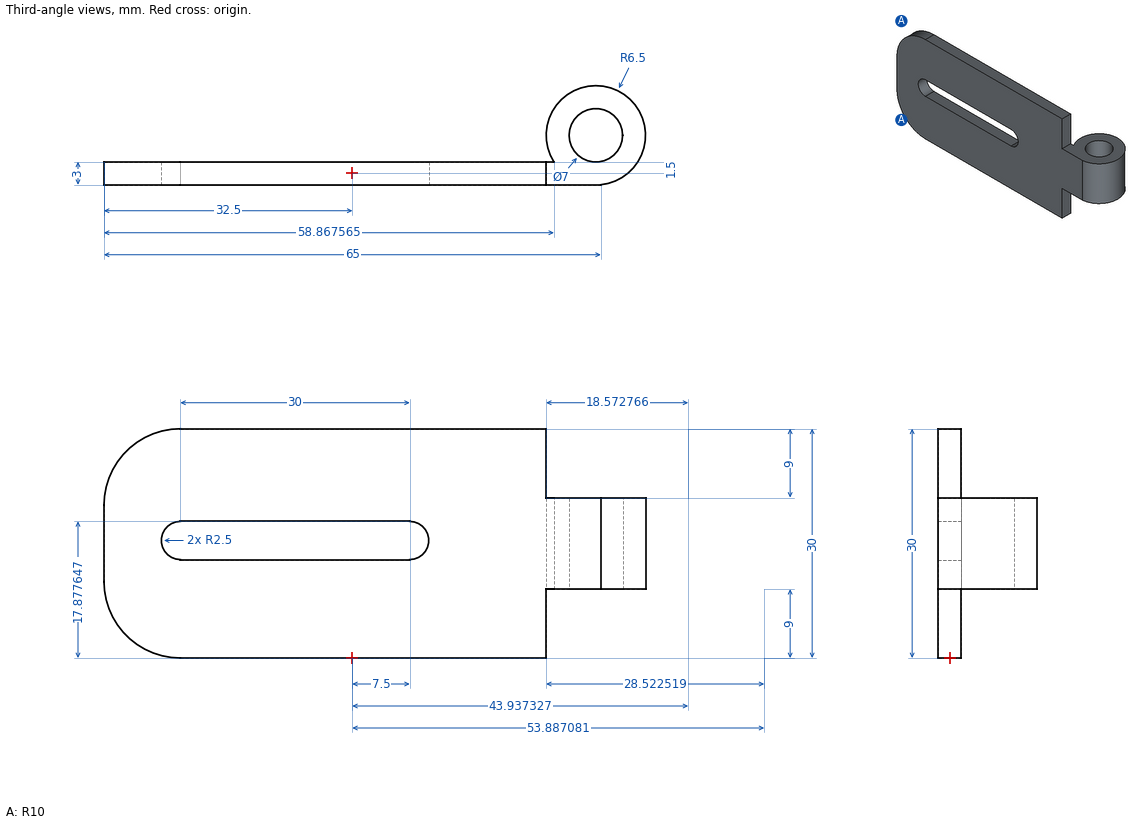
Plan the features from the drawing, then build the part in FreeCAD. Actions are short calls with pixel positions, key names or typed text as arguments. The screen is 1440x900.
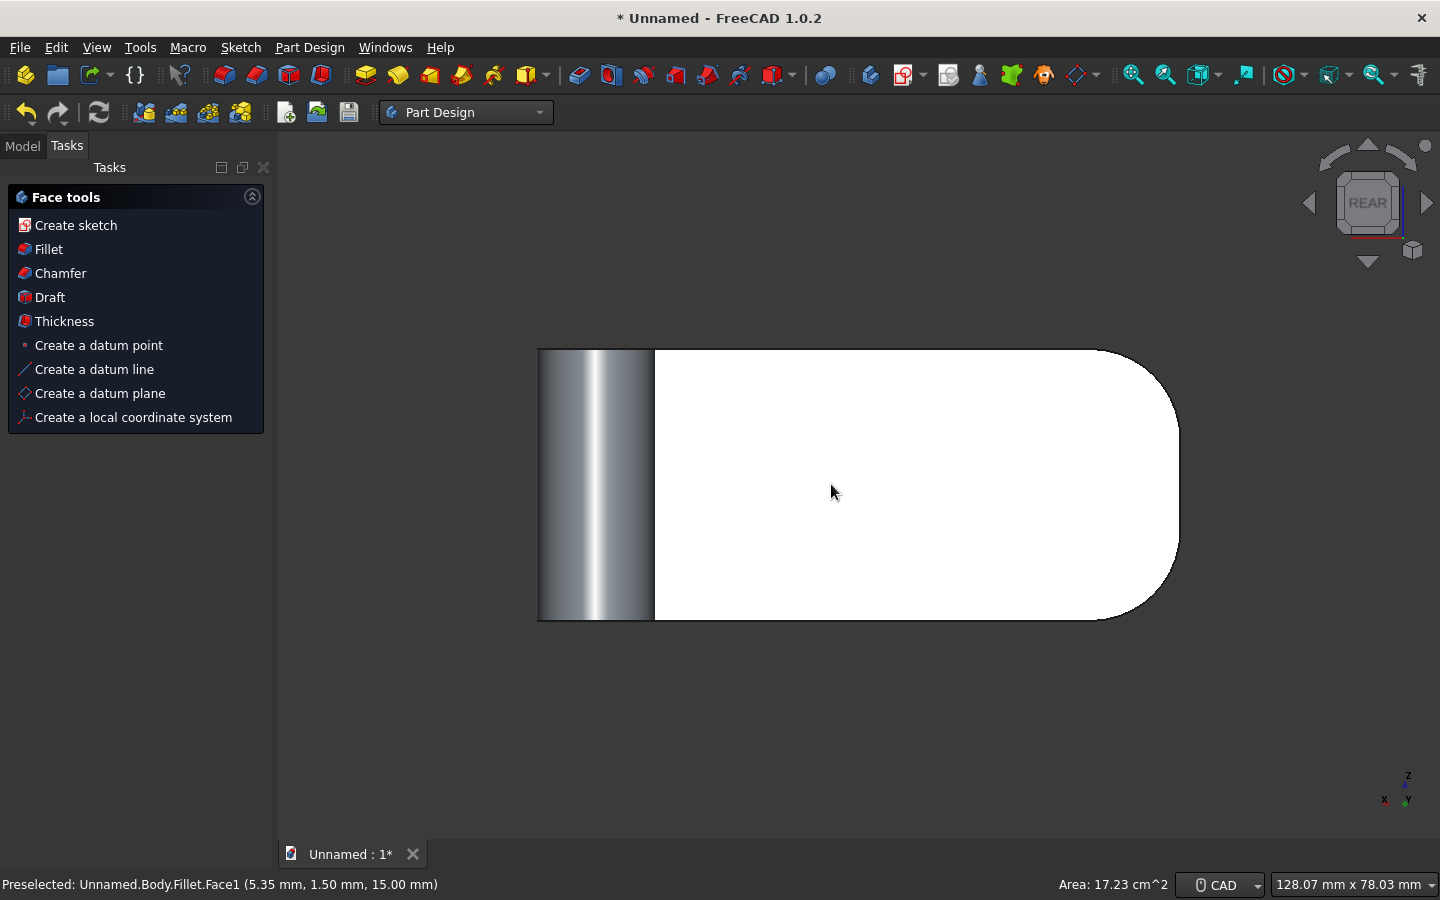
click(904, 76)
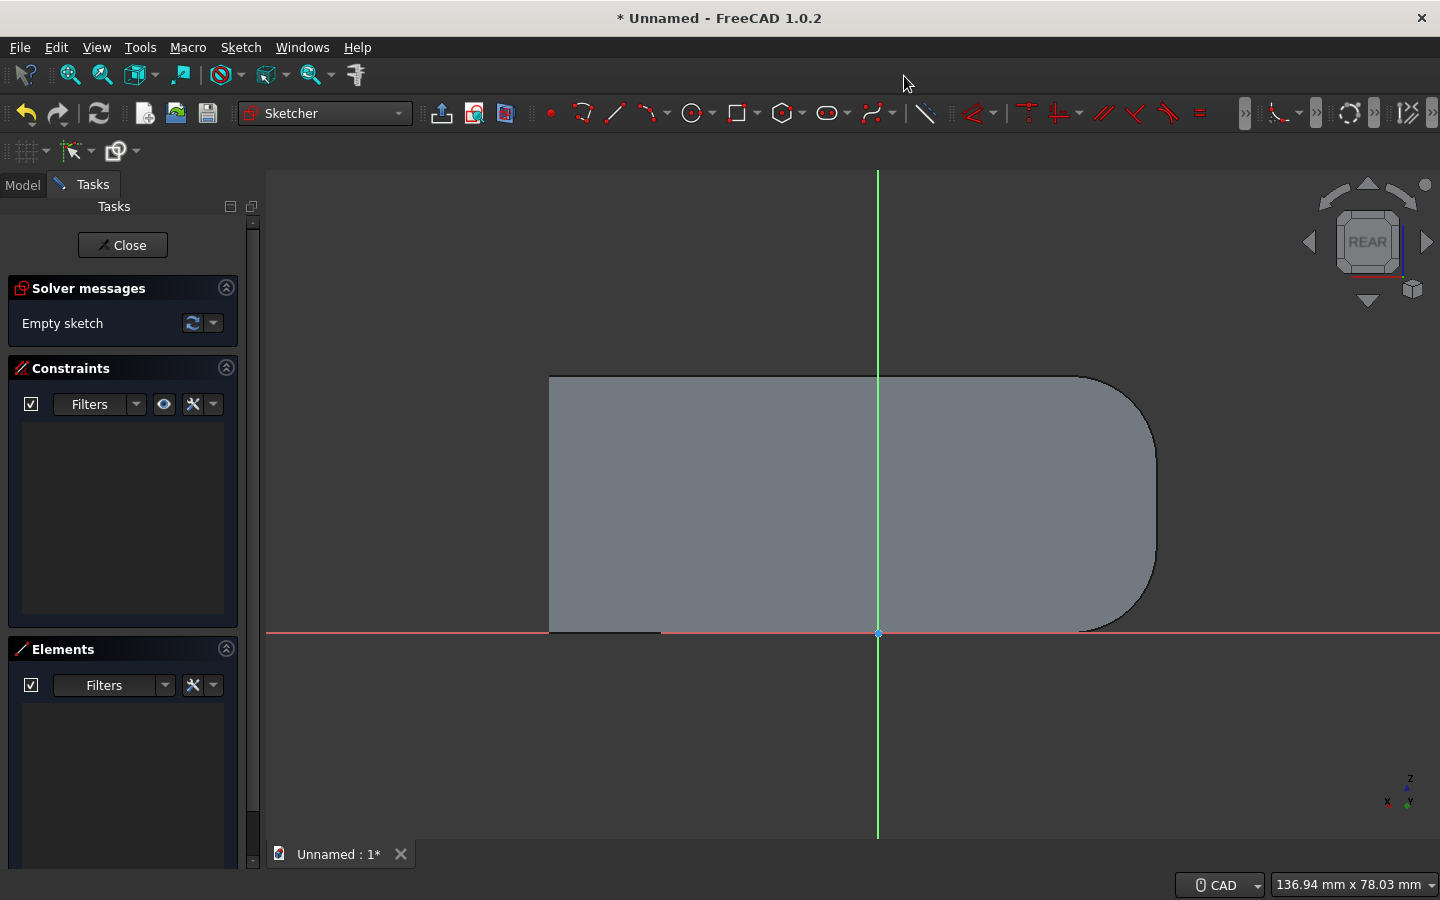
click(506, 114)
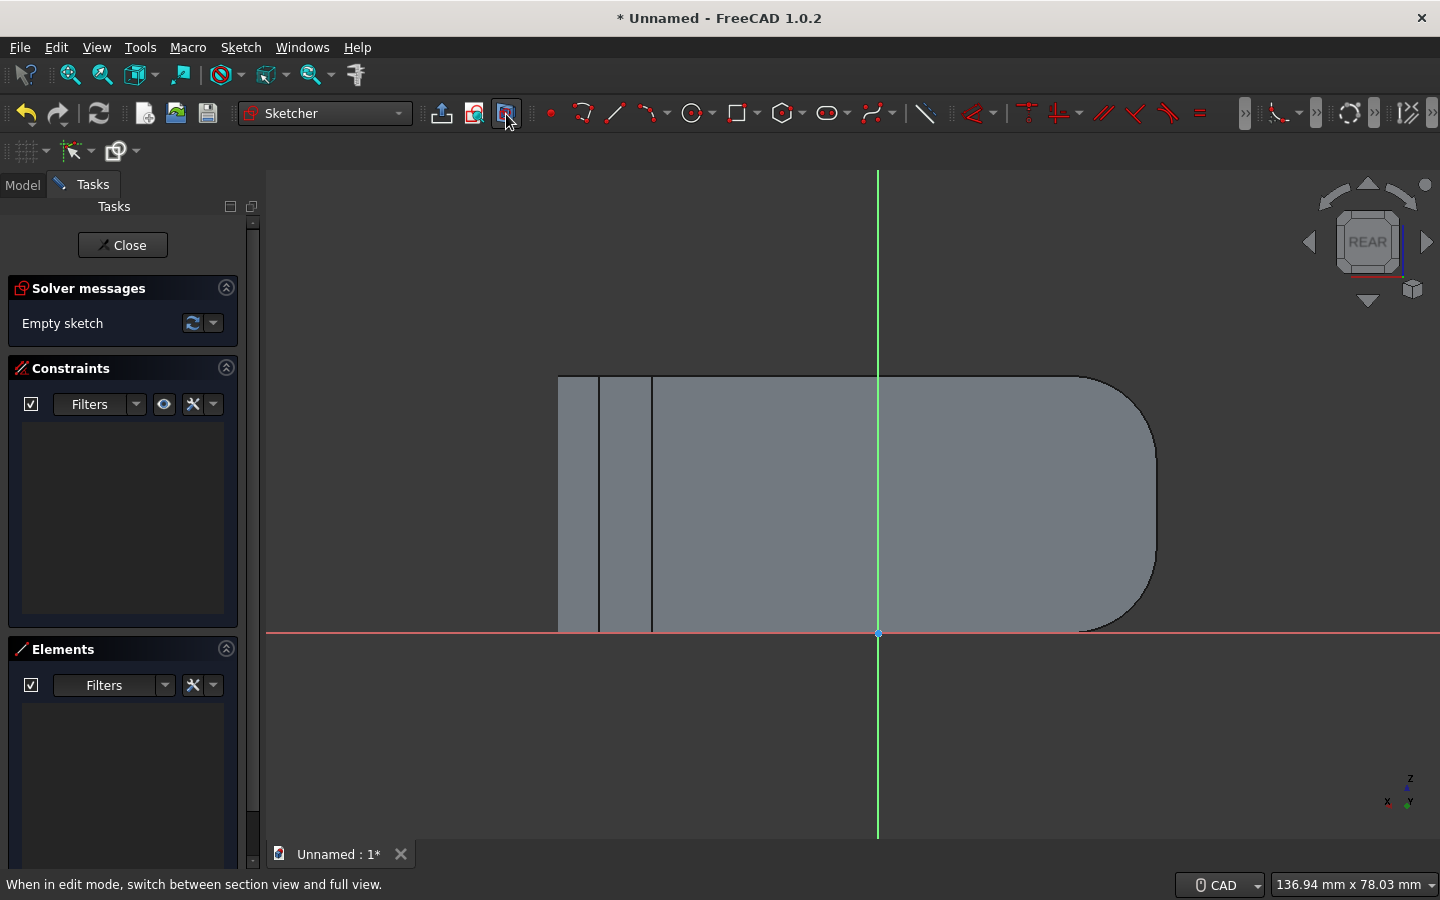
scroll(1071, 599, up, 4)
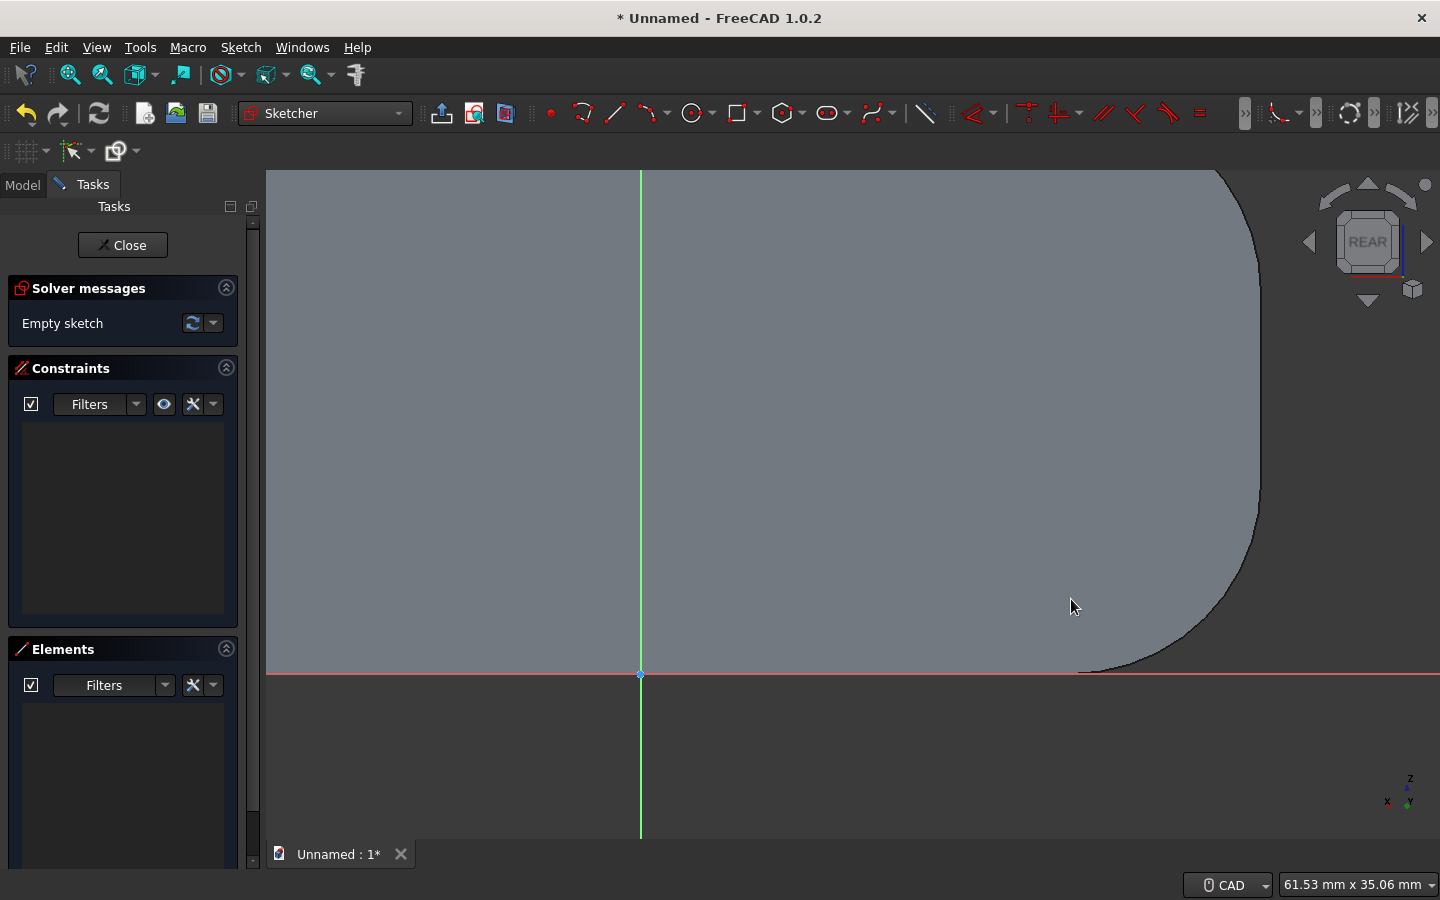
click(828, 114)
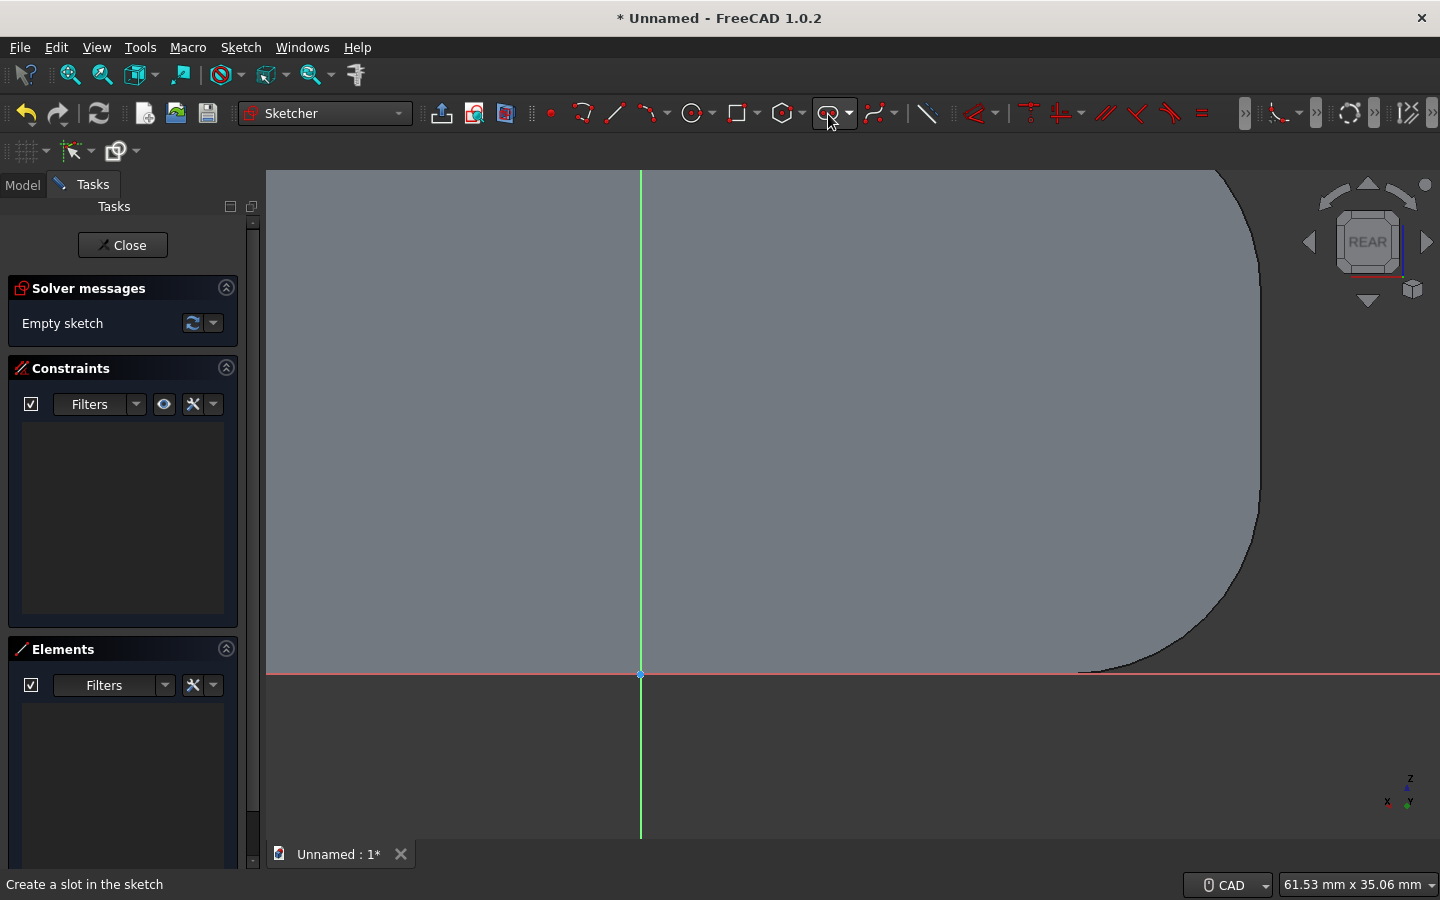
click(498, 381)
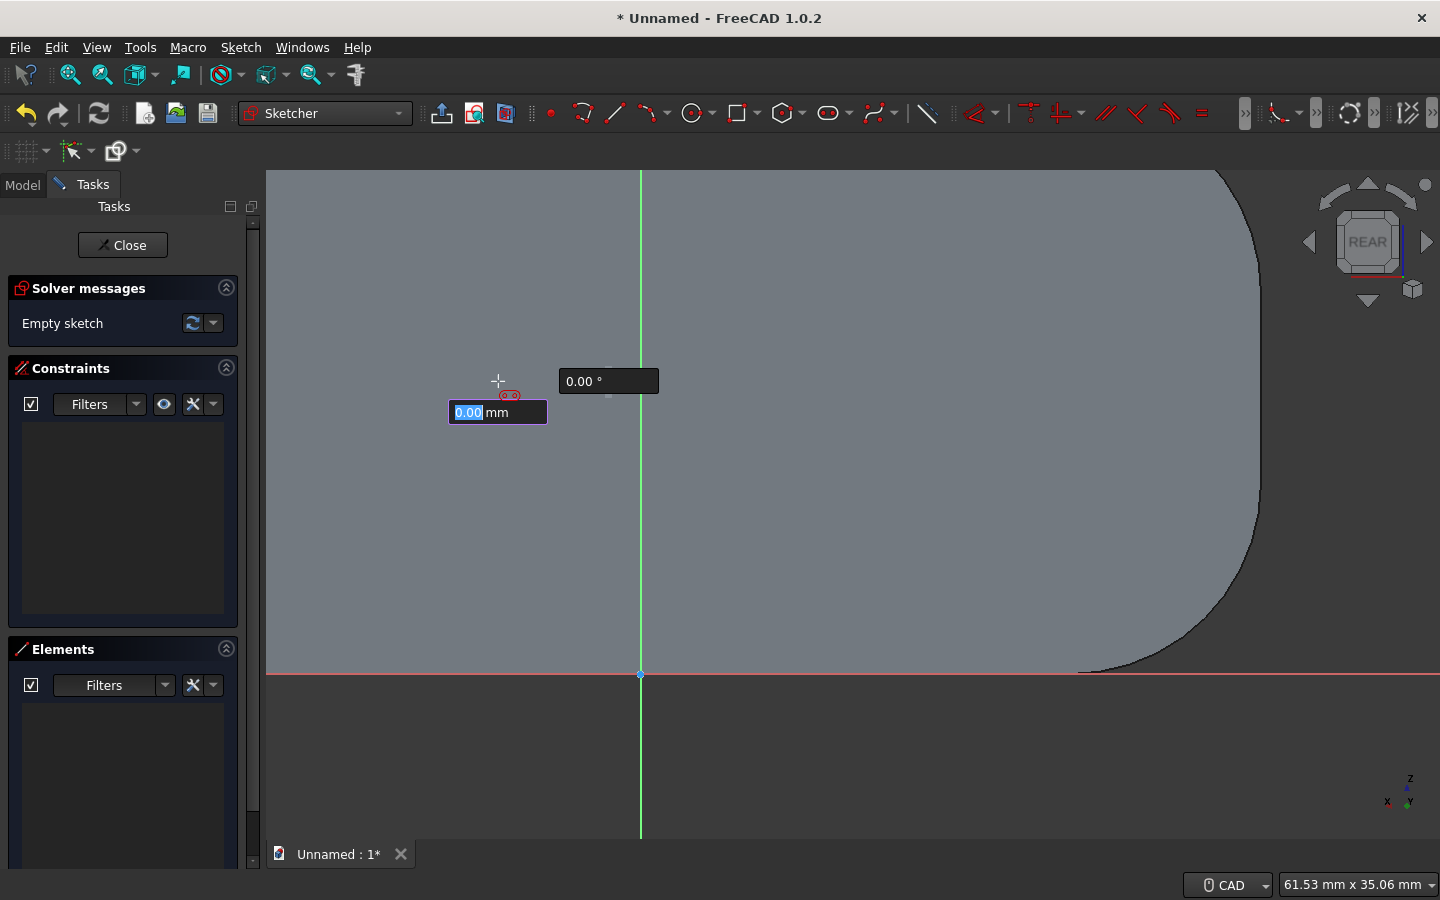
click(1070, 381)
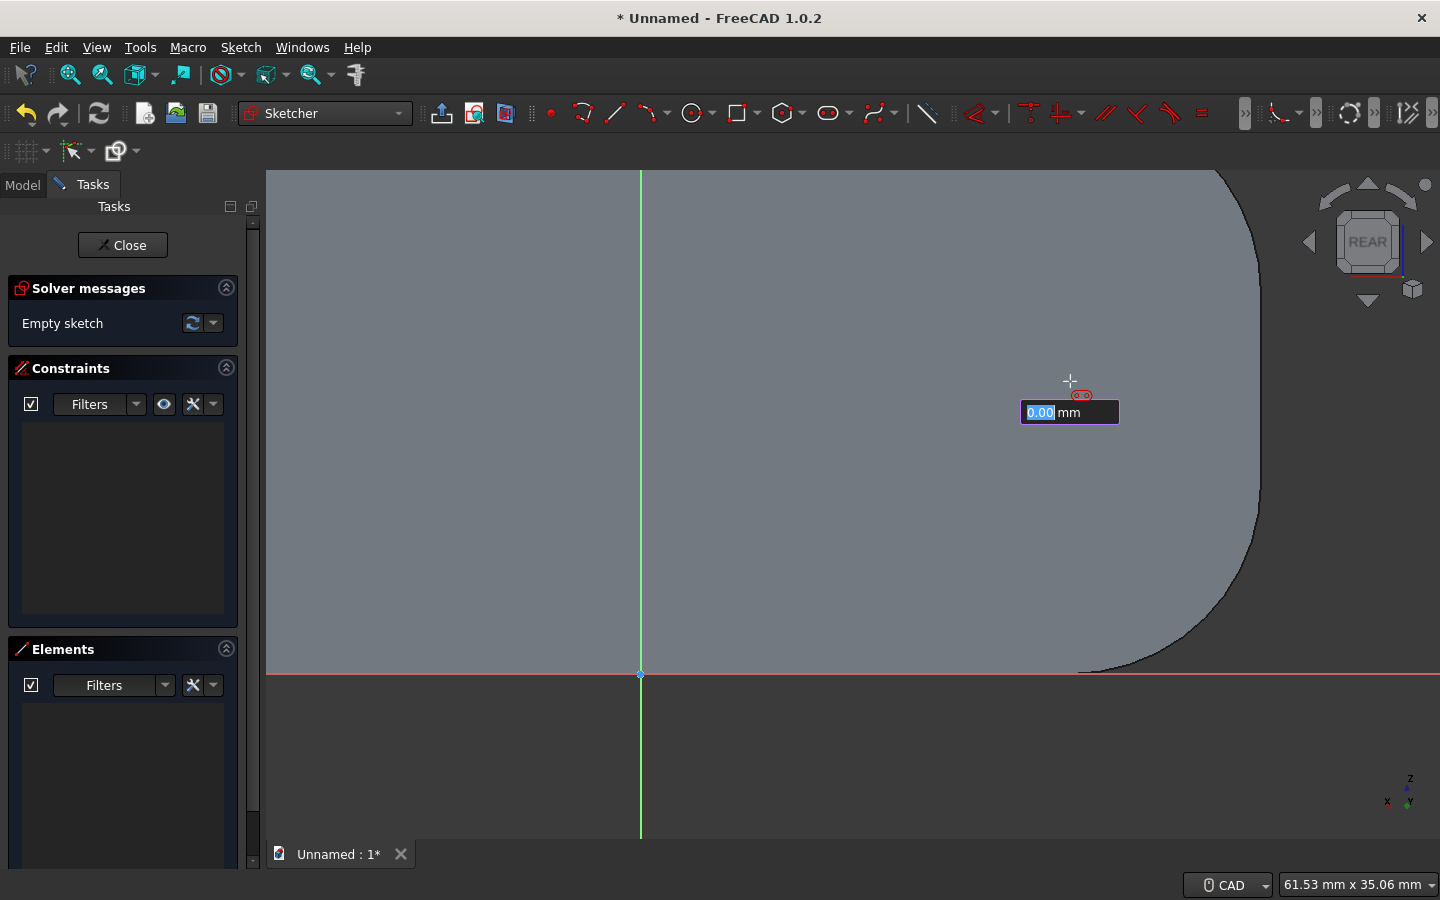
click(784, 428)
key(Escape)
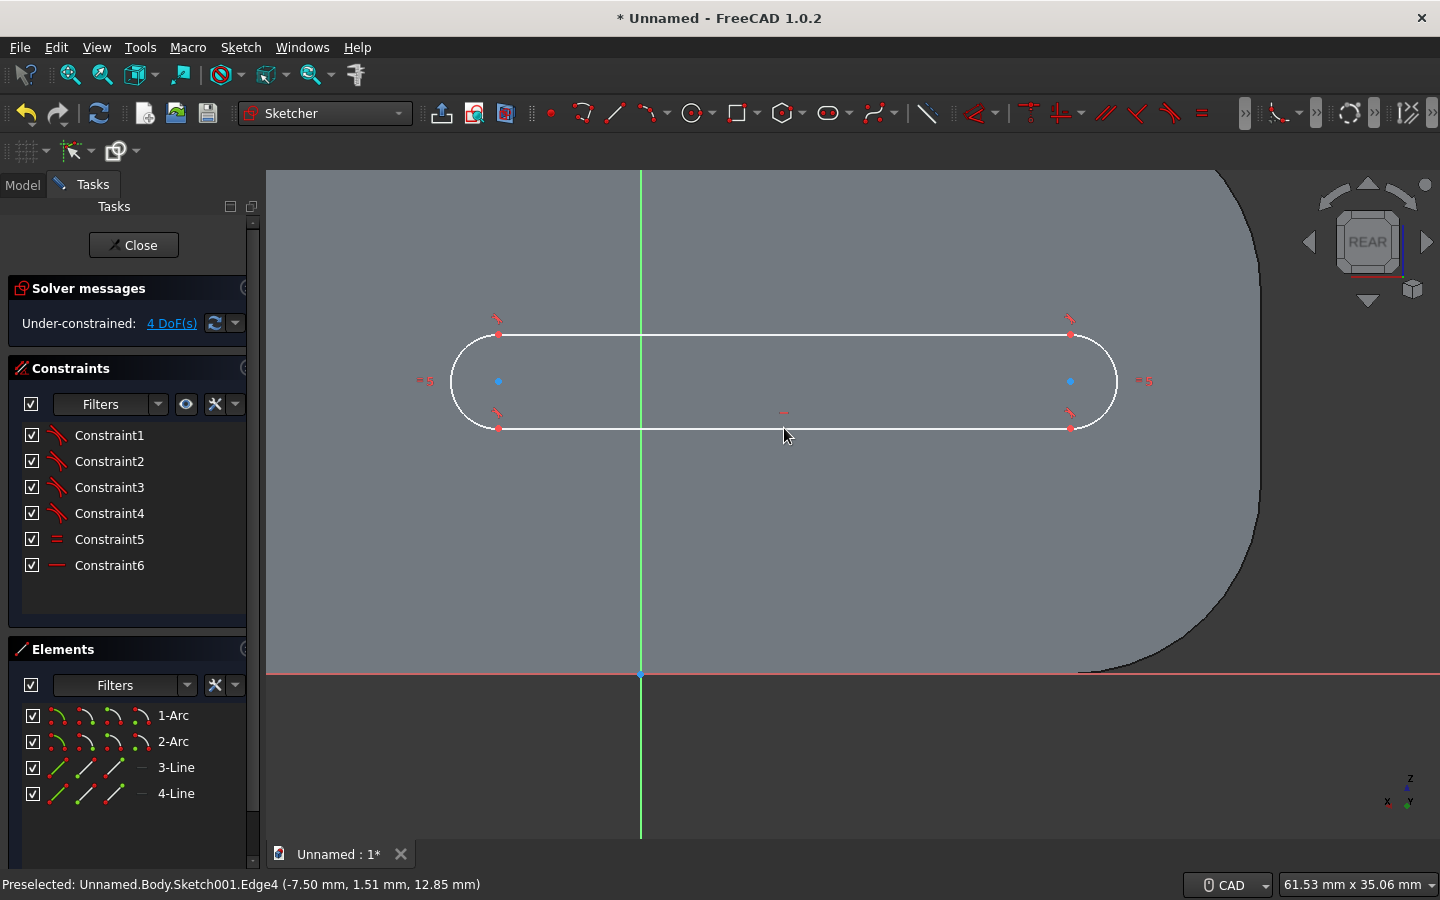
click(974, 114)